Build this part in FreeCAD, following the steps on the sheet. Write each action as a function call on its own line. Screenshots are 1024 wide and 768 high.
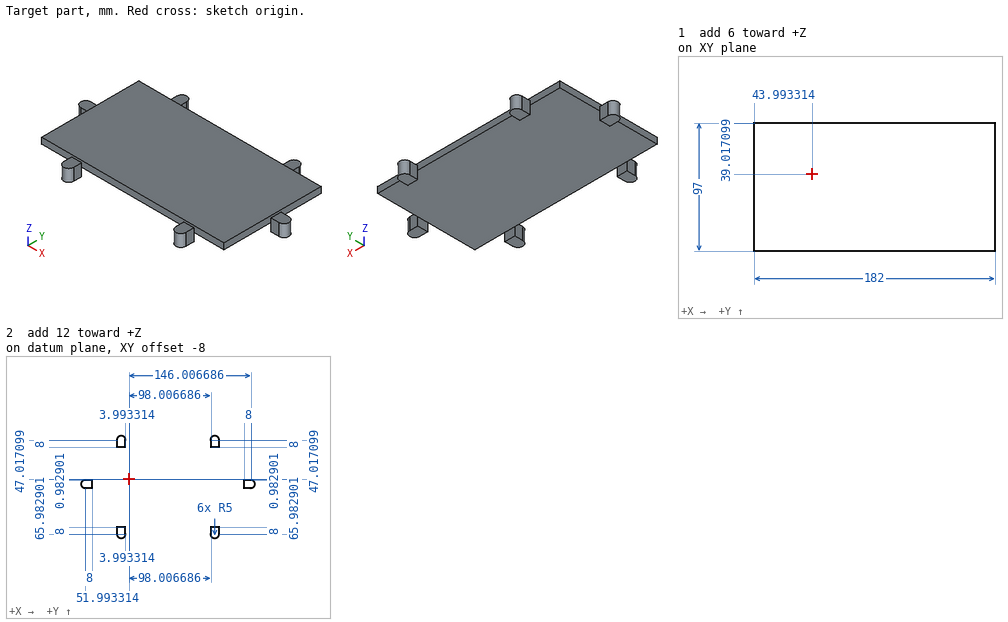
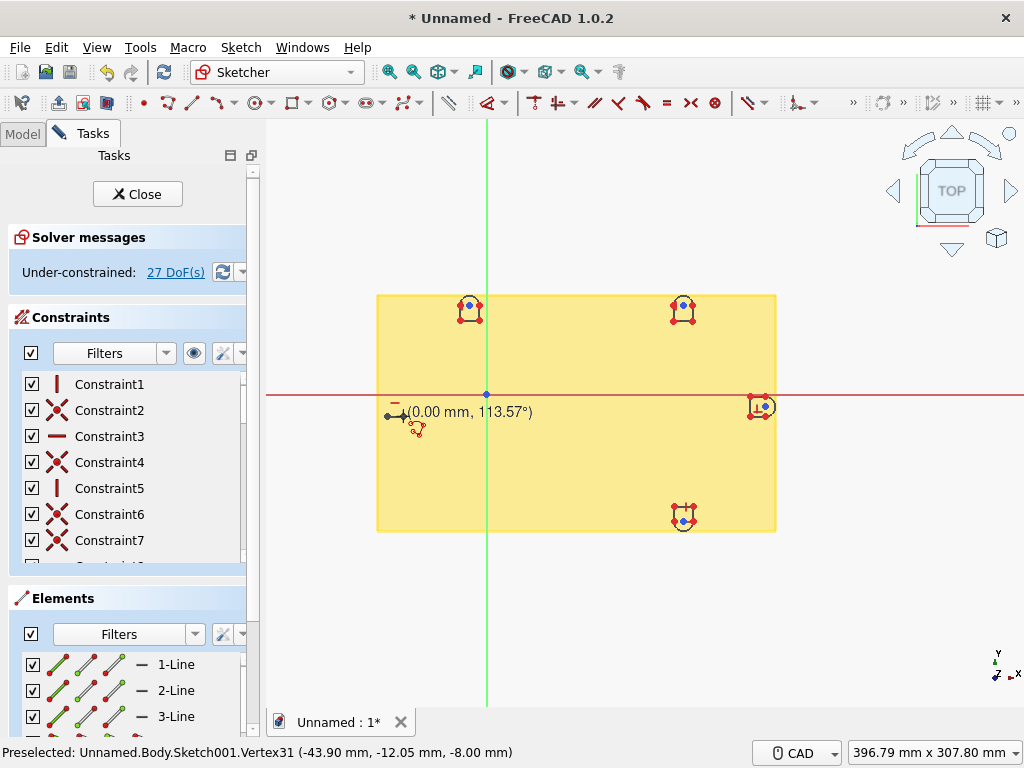
scroll(403, 397, up, 11)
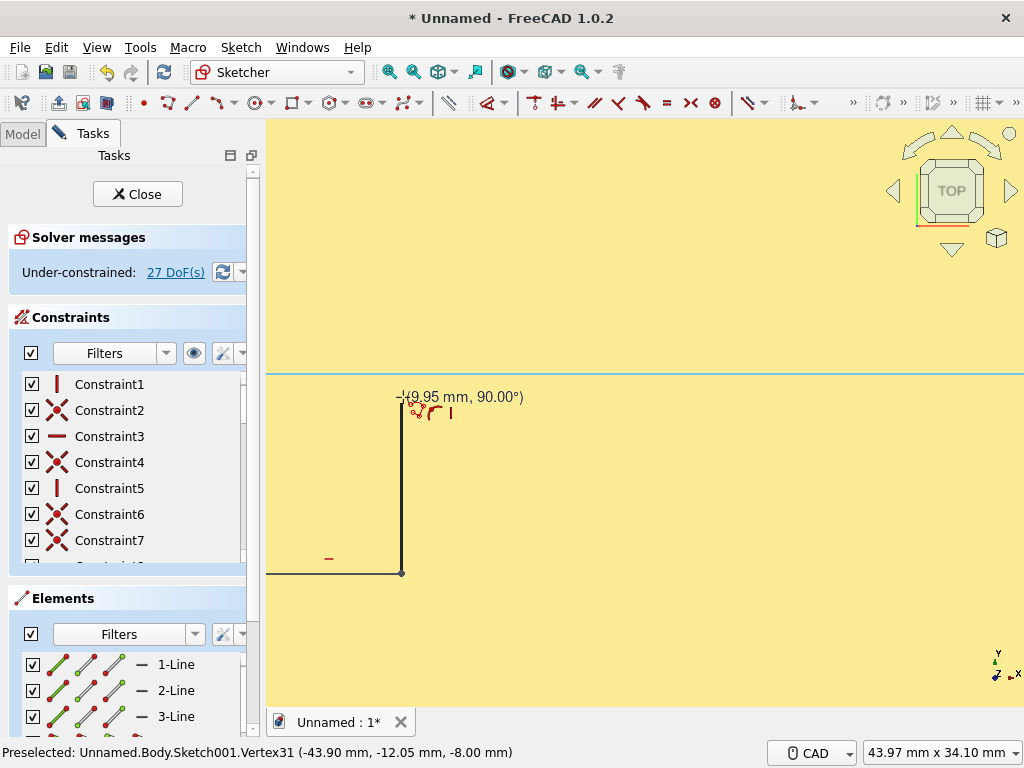
click(402, 391)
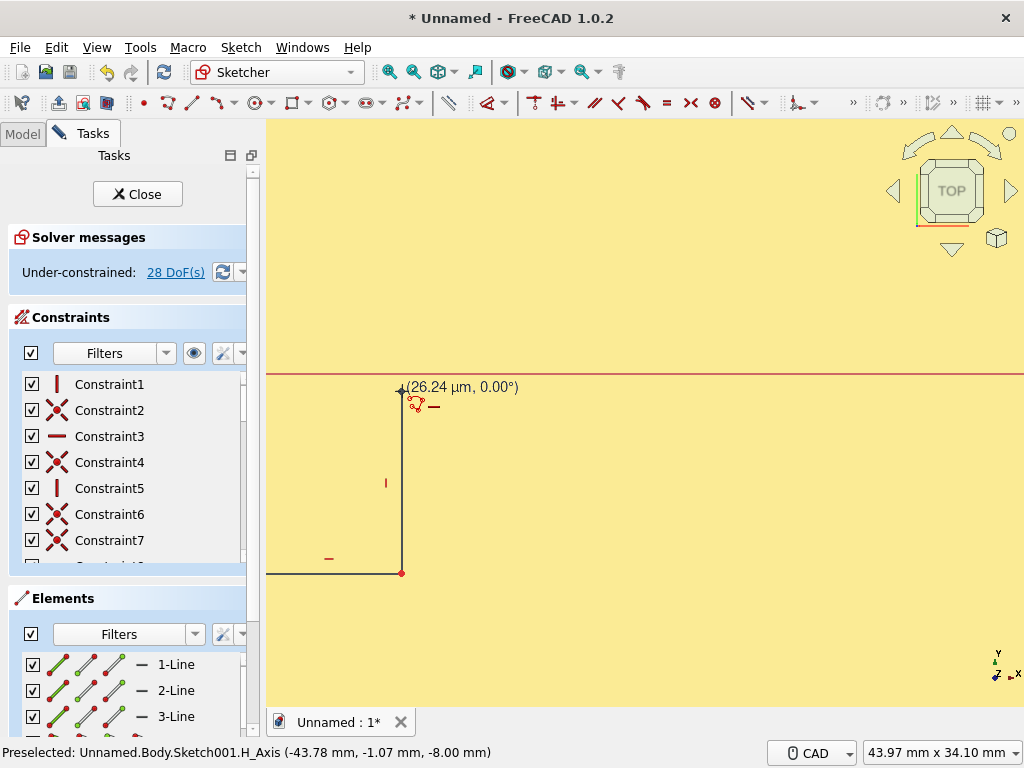
scroll(403, 397, down, 11)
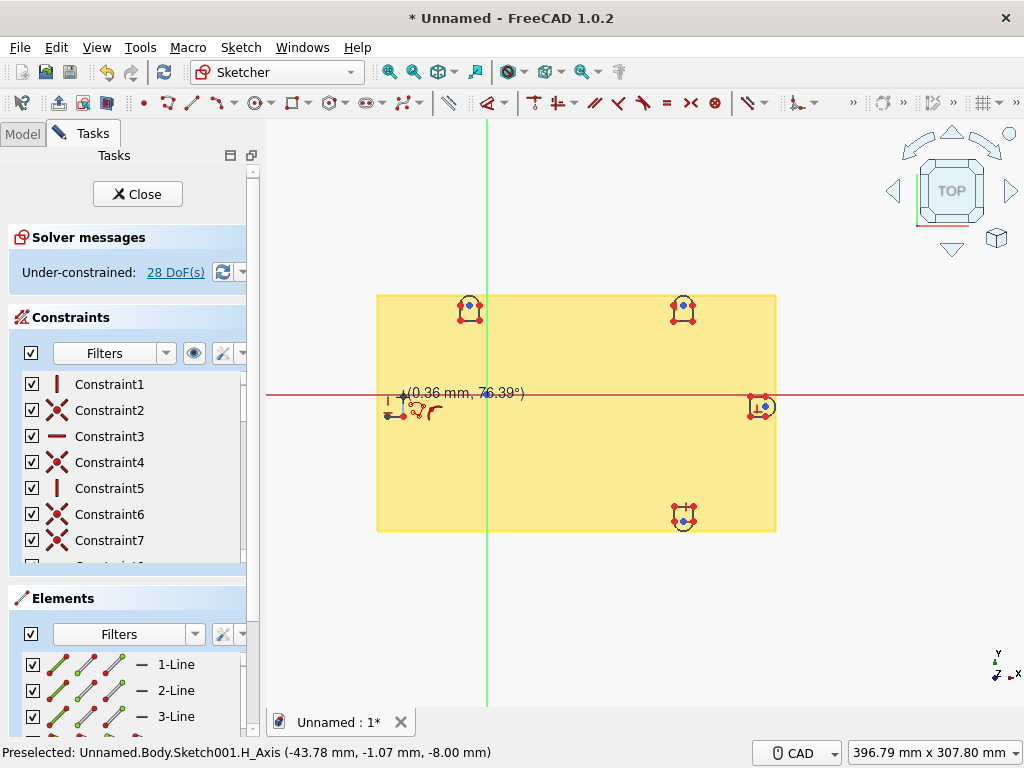
scroll(387, 397, up, 11)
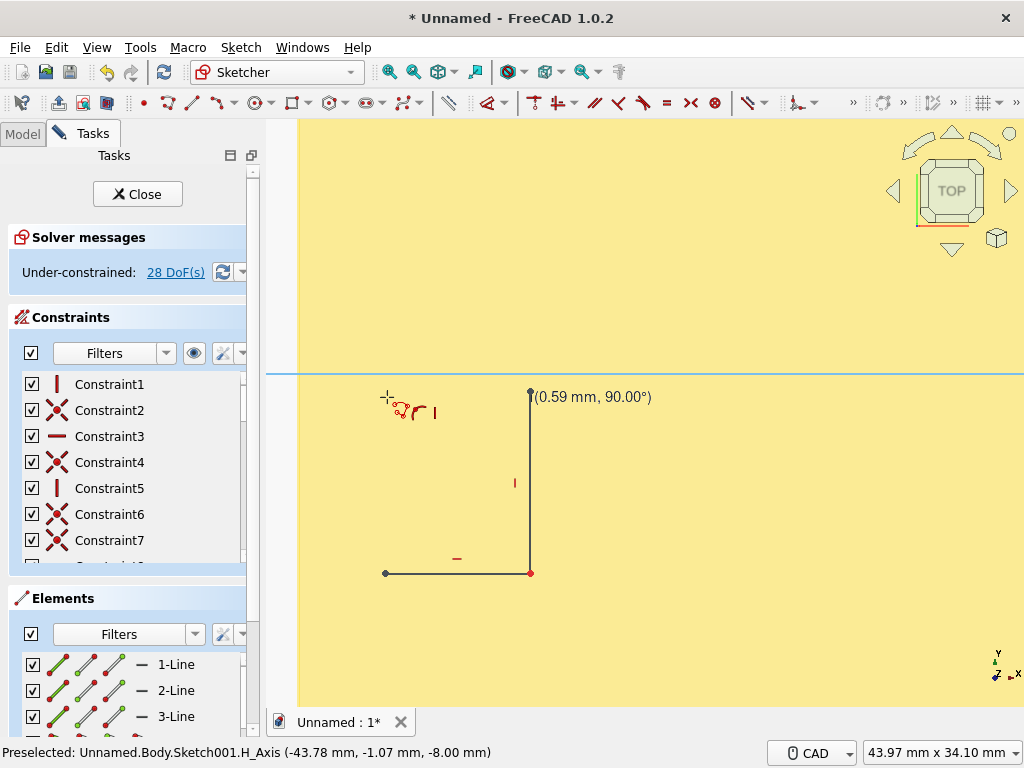
click(390, 391)
right_click(390, 391)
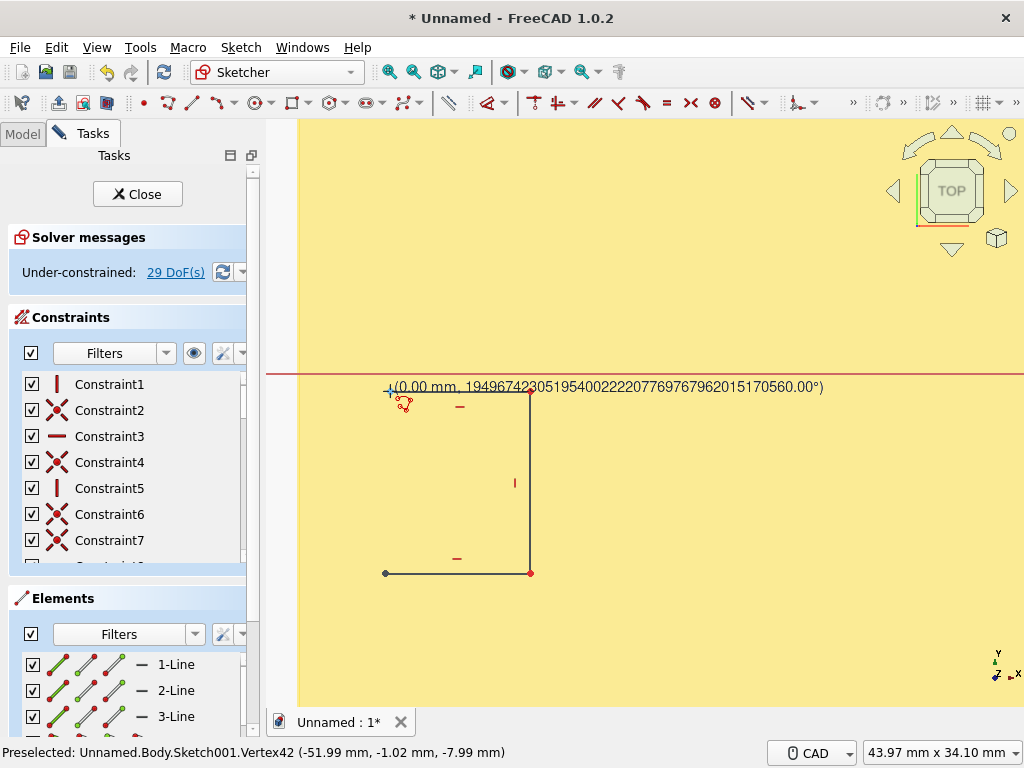
click(218, 104)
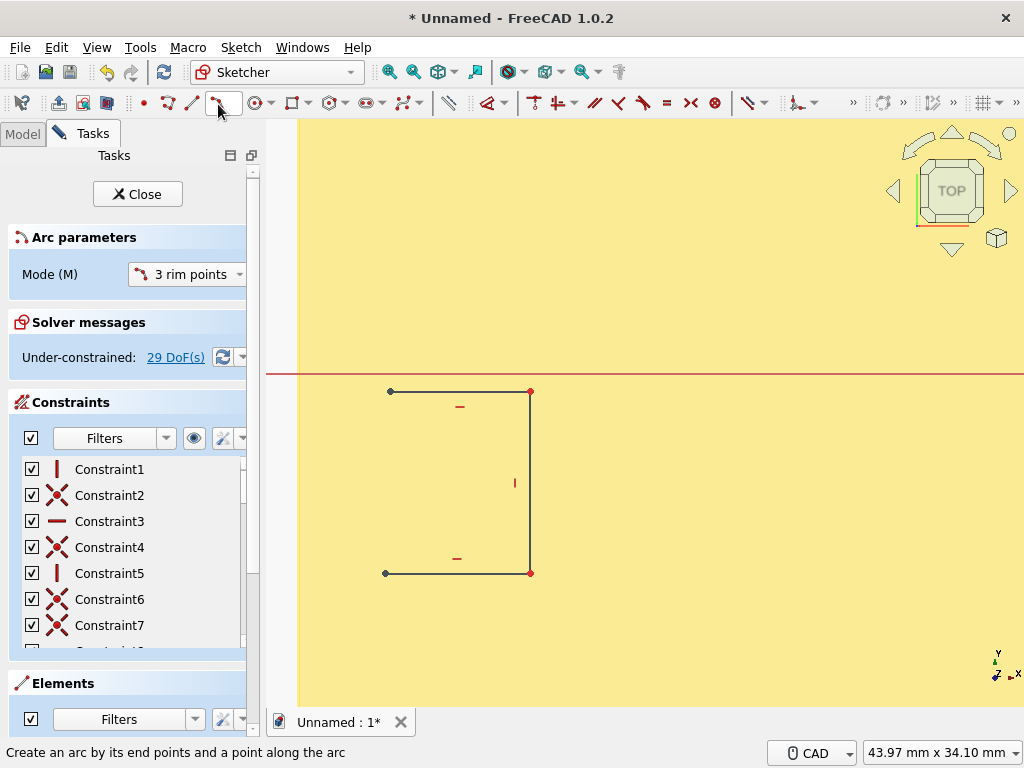
click(390, 392)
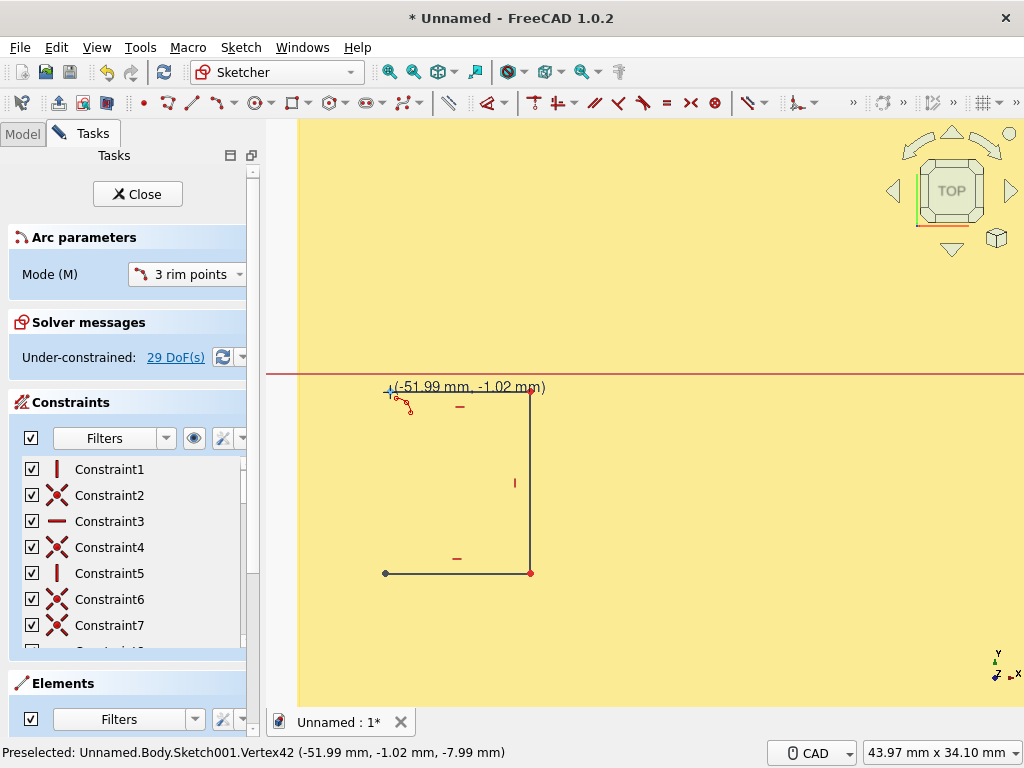
scroll(387, 397, down, 11)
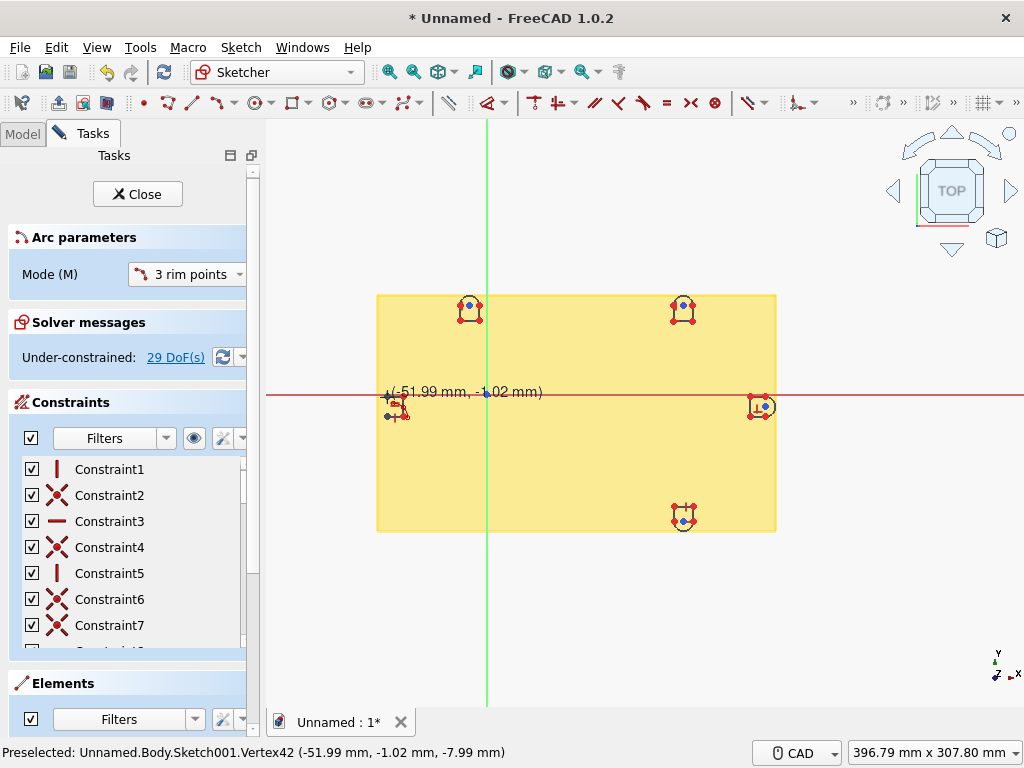
scroll(387, 416, up, 4)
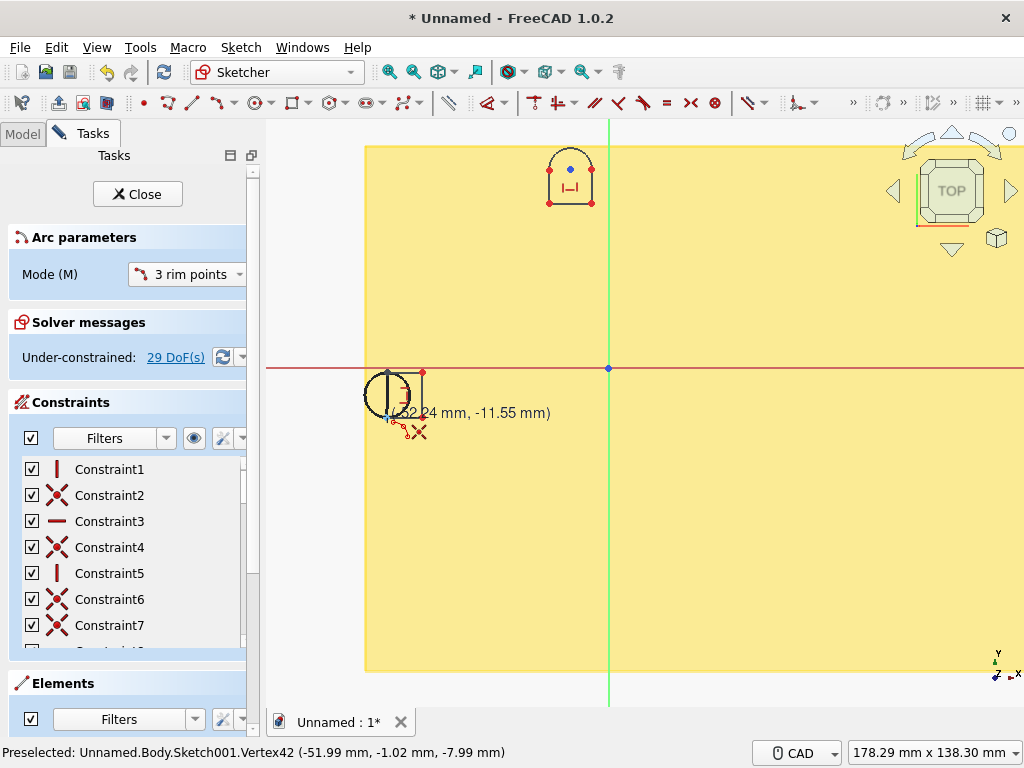
click(387, 418)
click(367, 394)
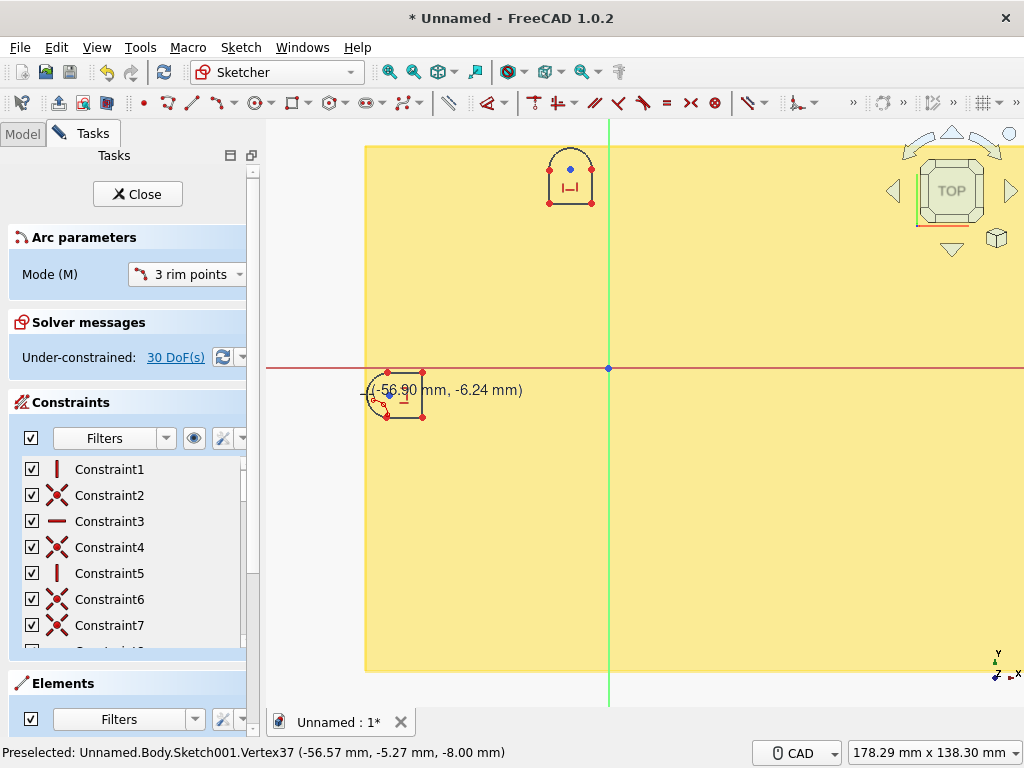
click(168, 104)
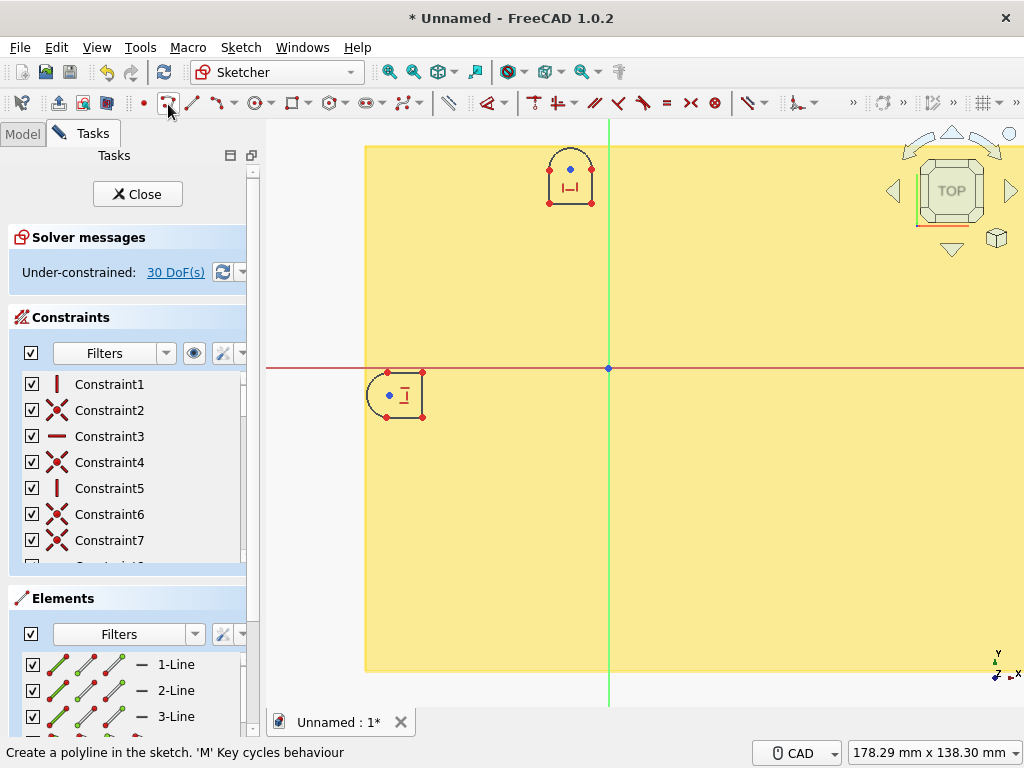
click(592, 649)
click(592, 615)
click(549, 615)
click(549, 649)
right_click(549, 649)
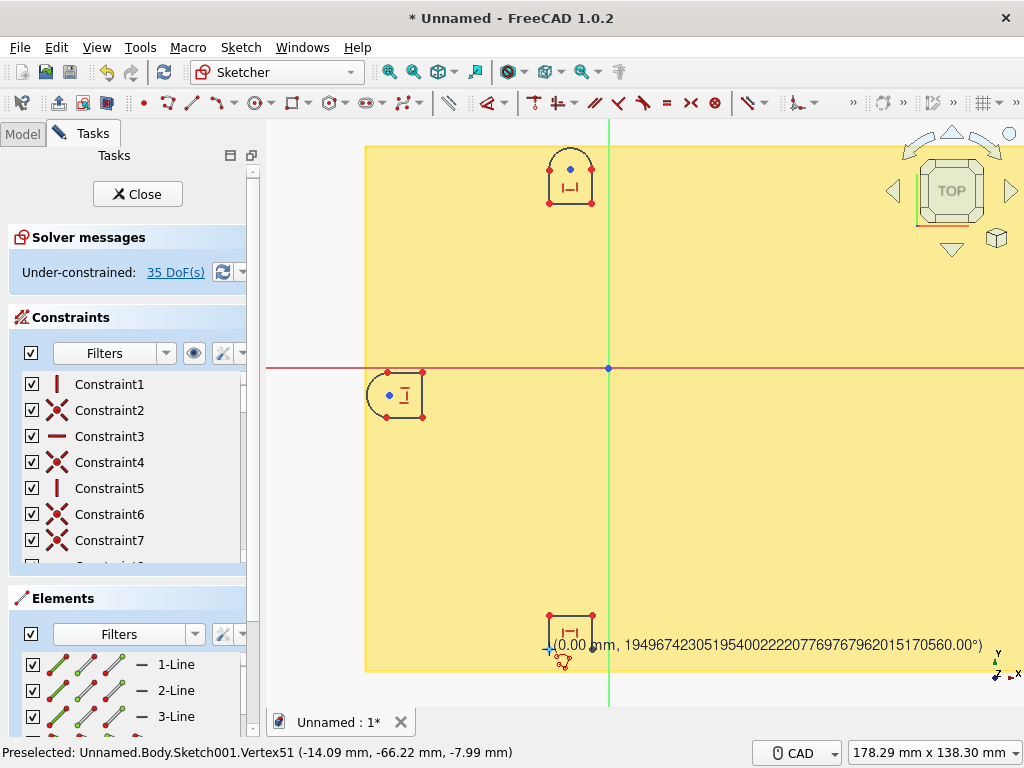
click(218, 104)